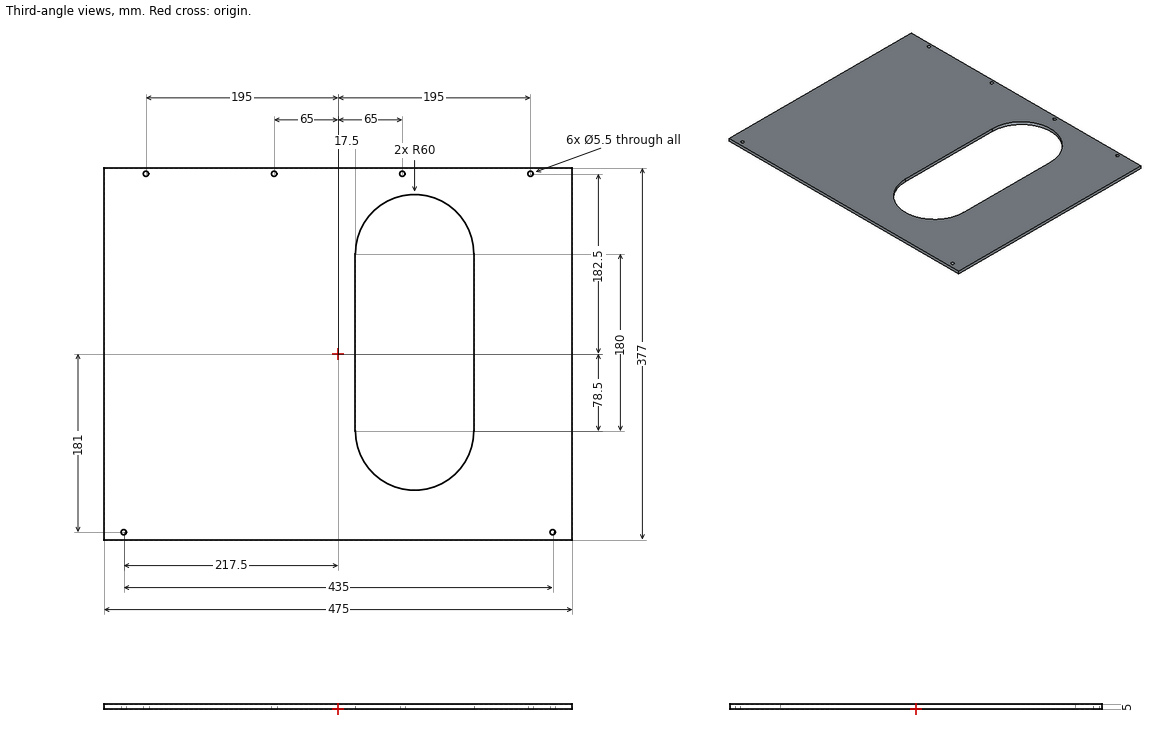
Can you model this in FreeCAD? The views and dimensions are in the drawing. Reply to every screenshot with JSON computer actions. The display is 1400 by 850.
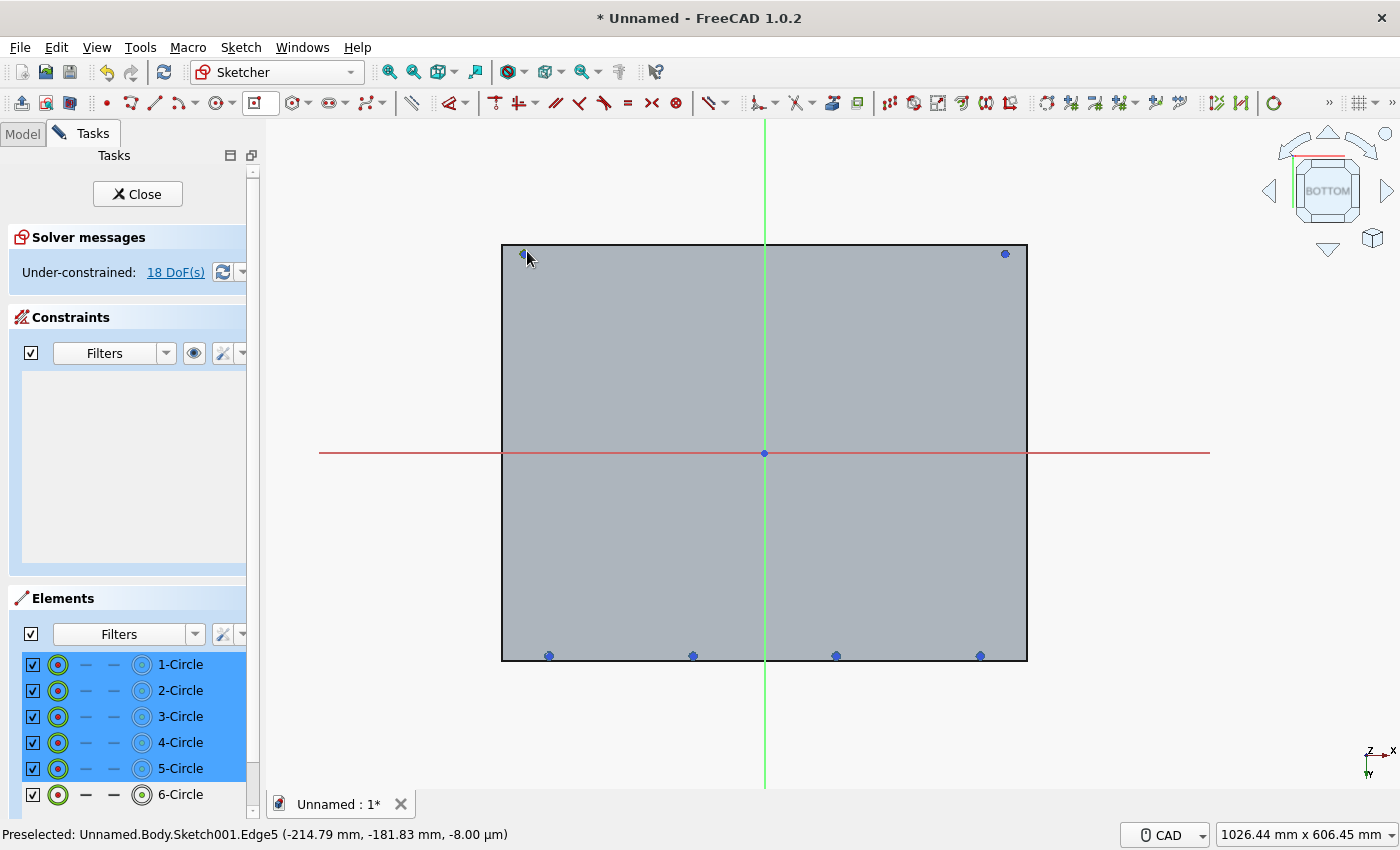
{"action": "scroll", "coordinate": [1008, 252], "scroll_direction": "up", "scroll_amount": 7}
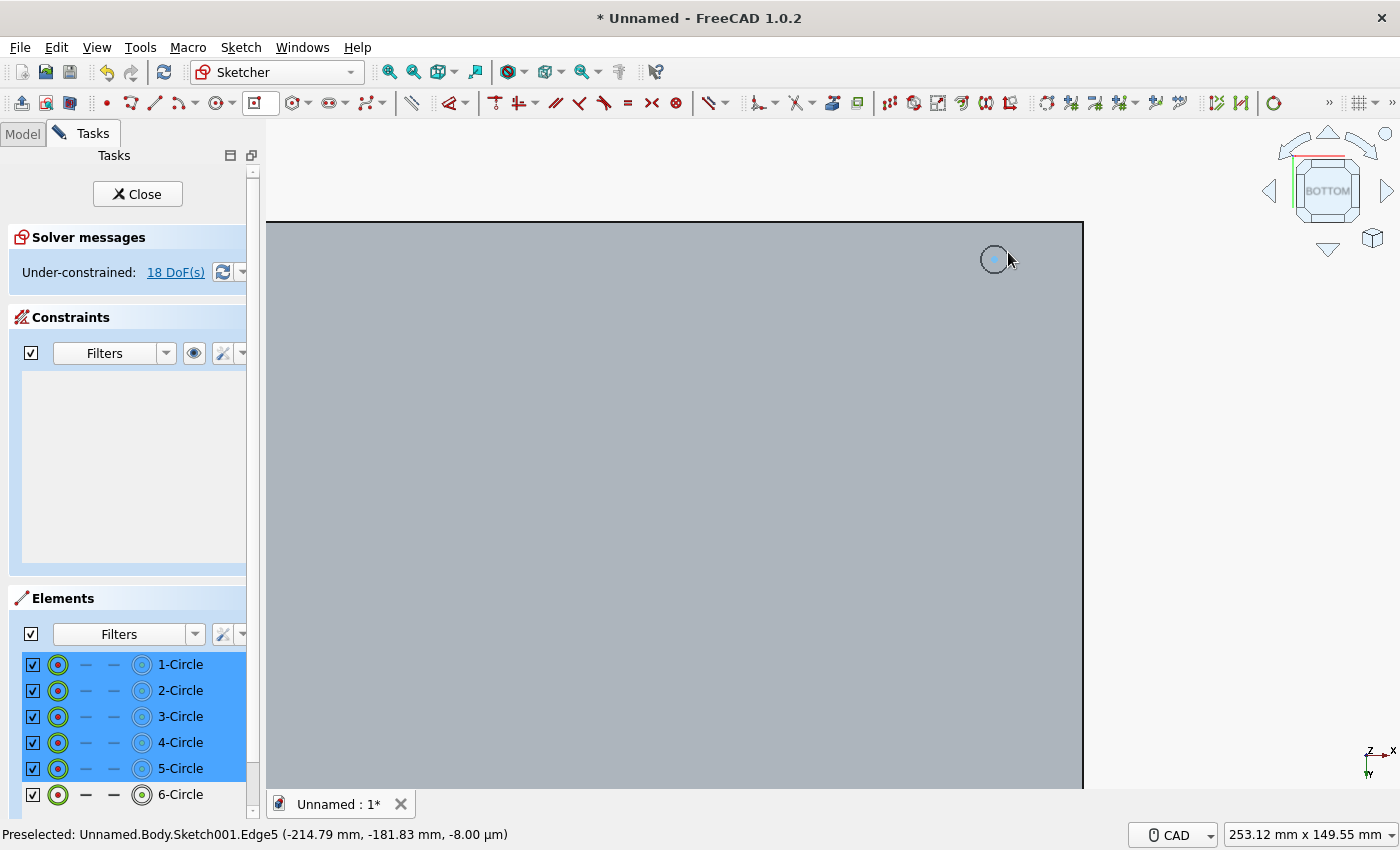
{"action": "left_click", "coordinate": [1005, 250]}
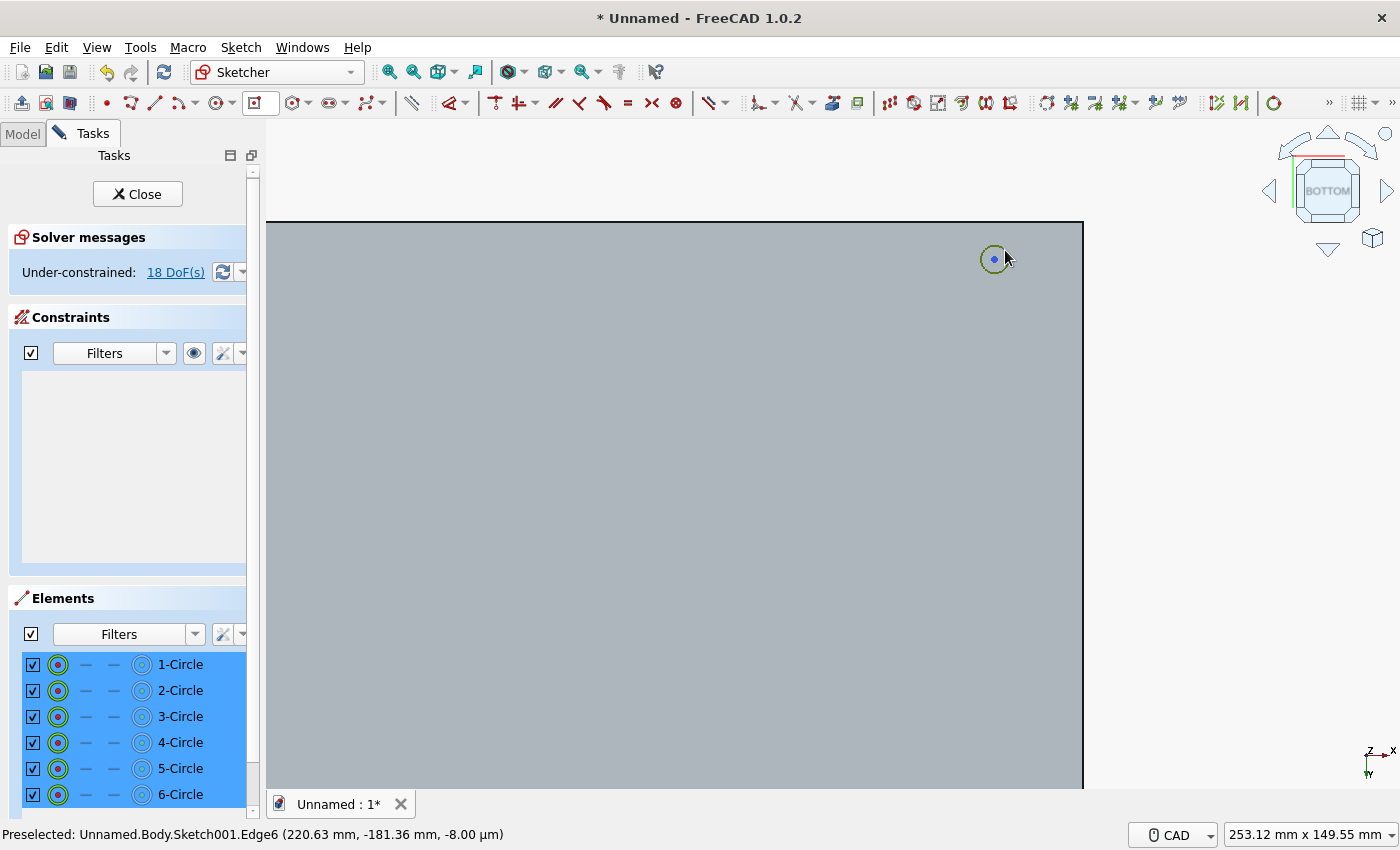
{"action": "key", "text": "e"}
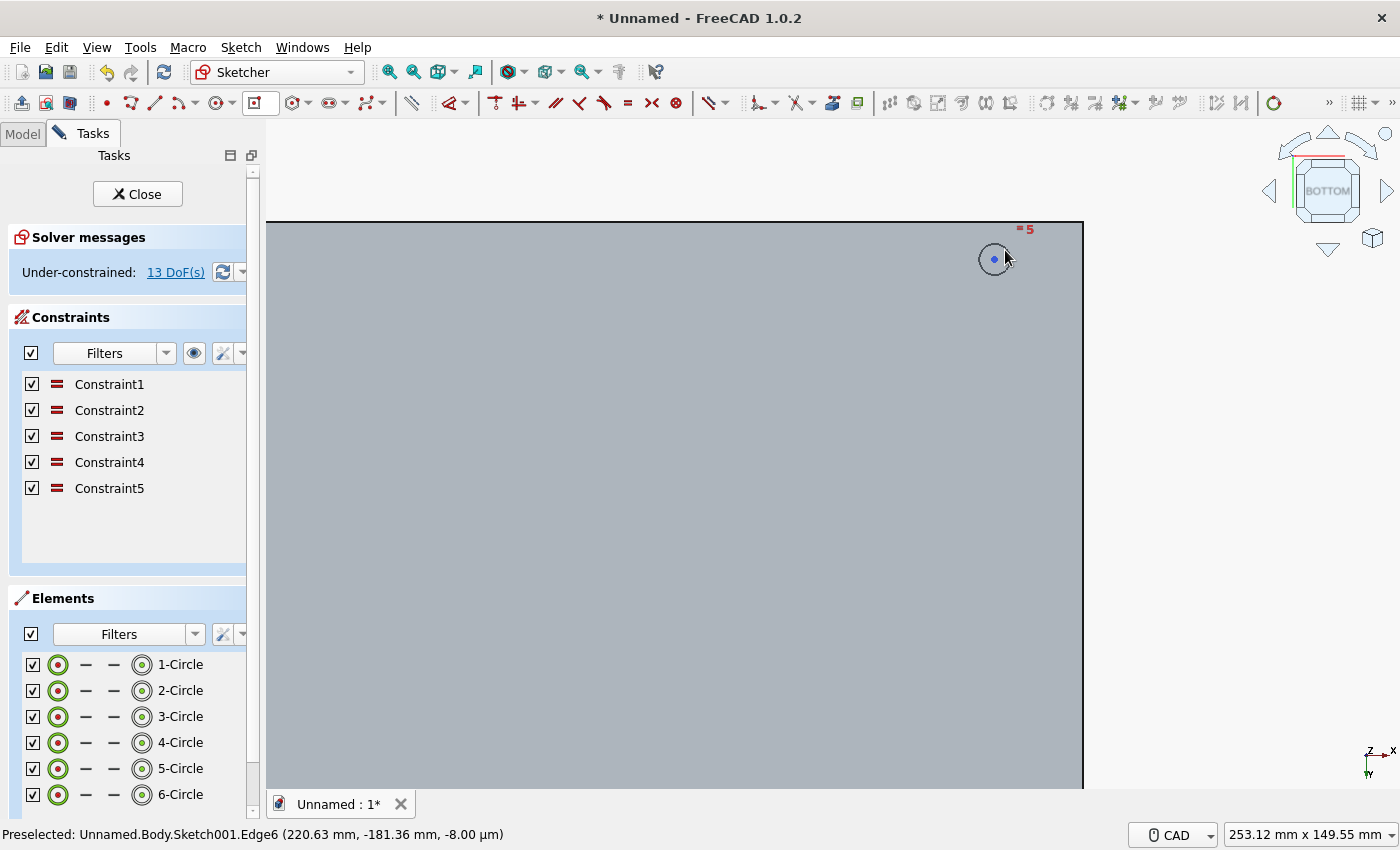
{"action": "scroll", "coordinate": [1008, 252], "scroll_direction": "down", "scroll_amount": 7}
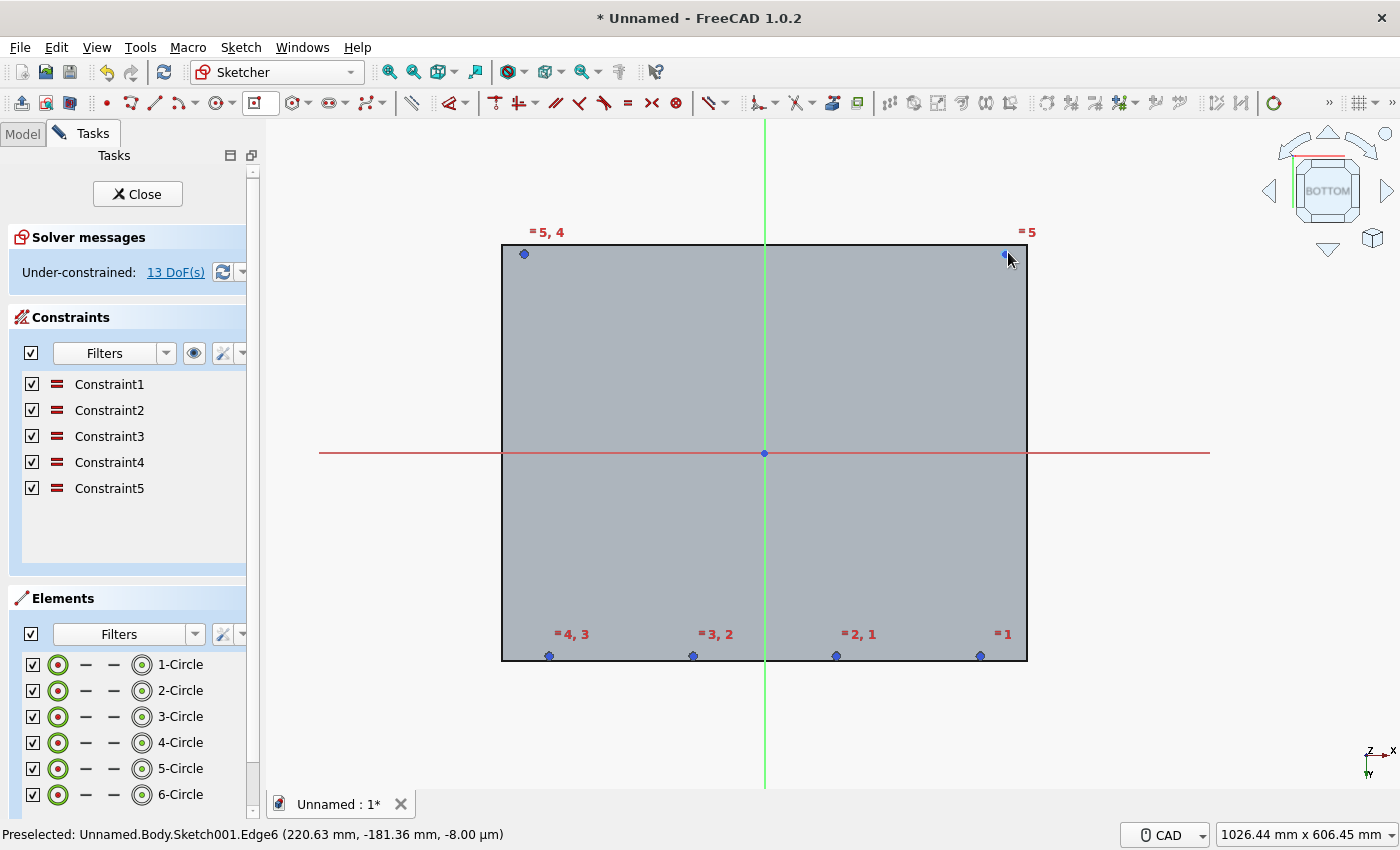
{"action": "left_click", "coordinate": [980, 656]}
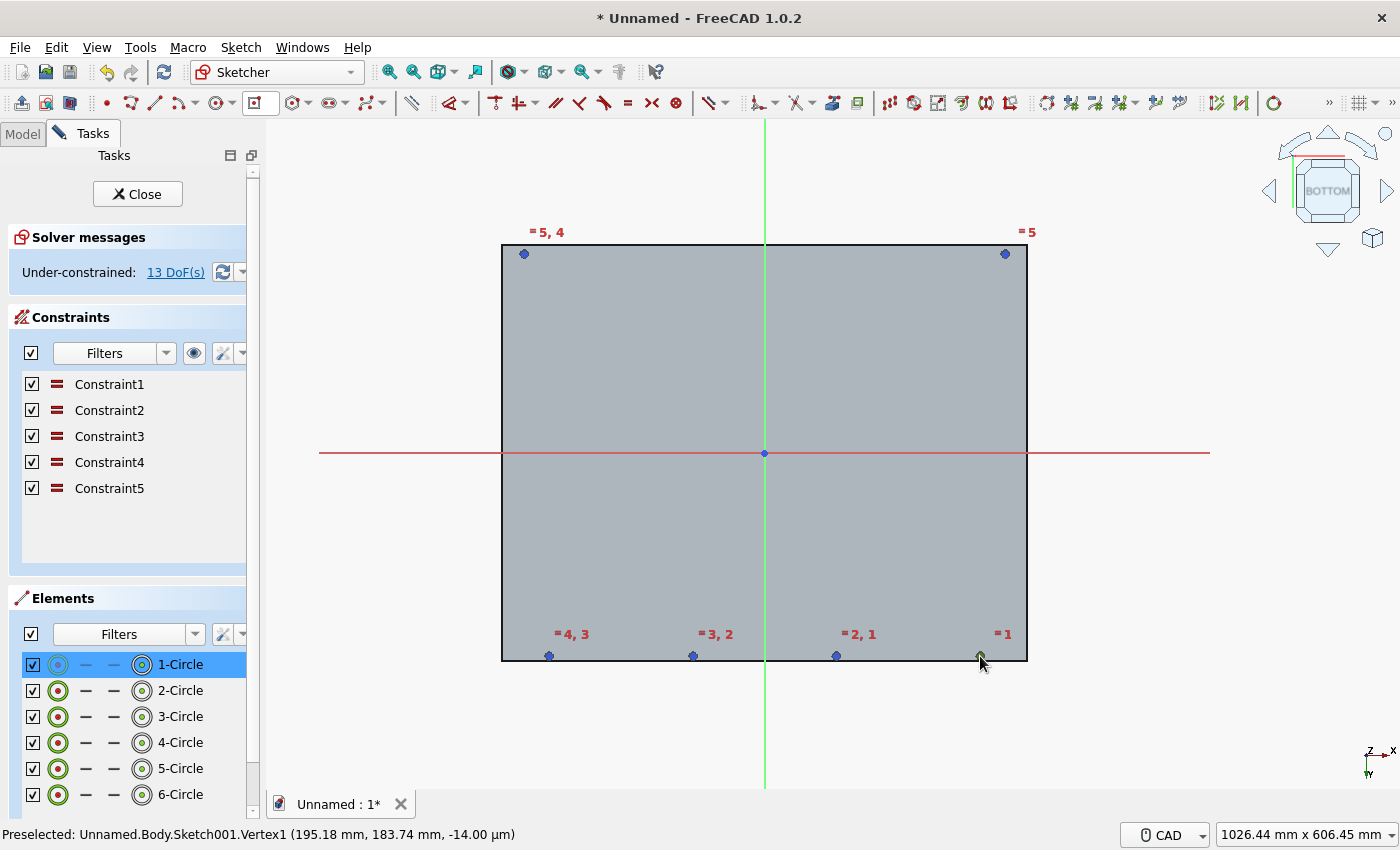
{"action": "left_click", "coordinate": [836, 656]}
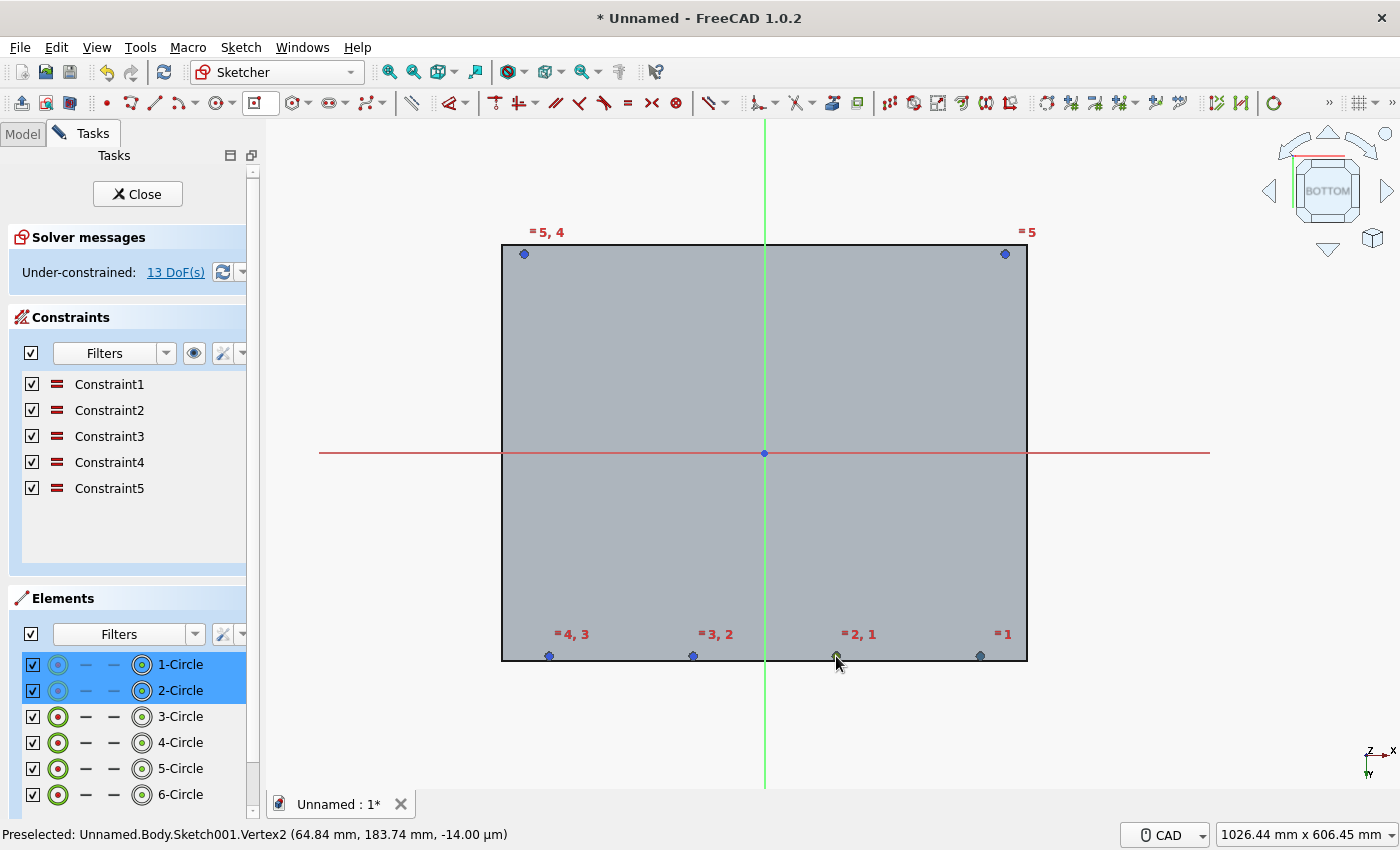
{"action": "left_click", "coordinate": [538, 104]}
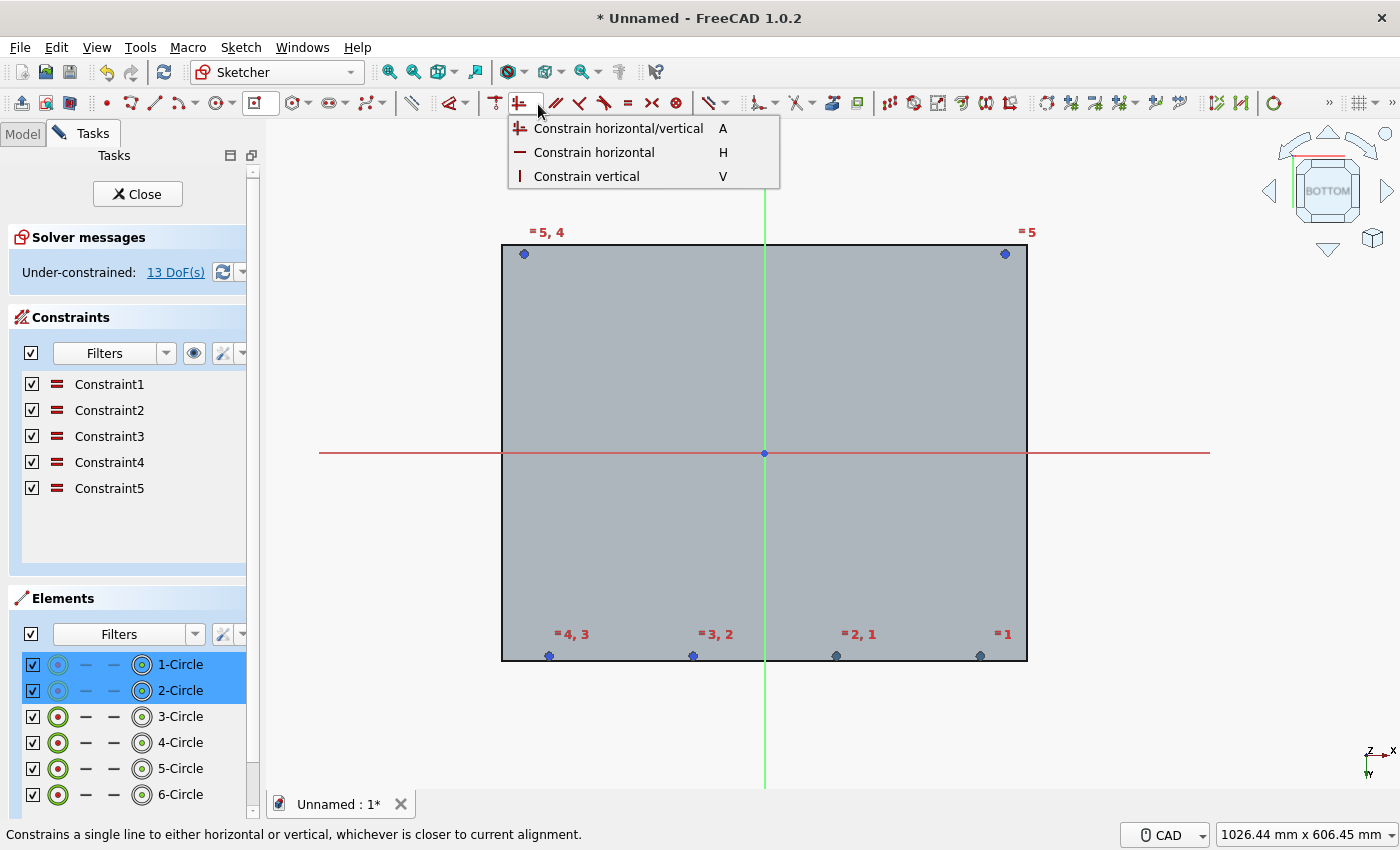
{"action": "left_click", "coordinate": [644, 152]}